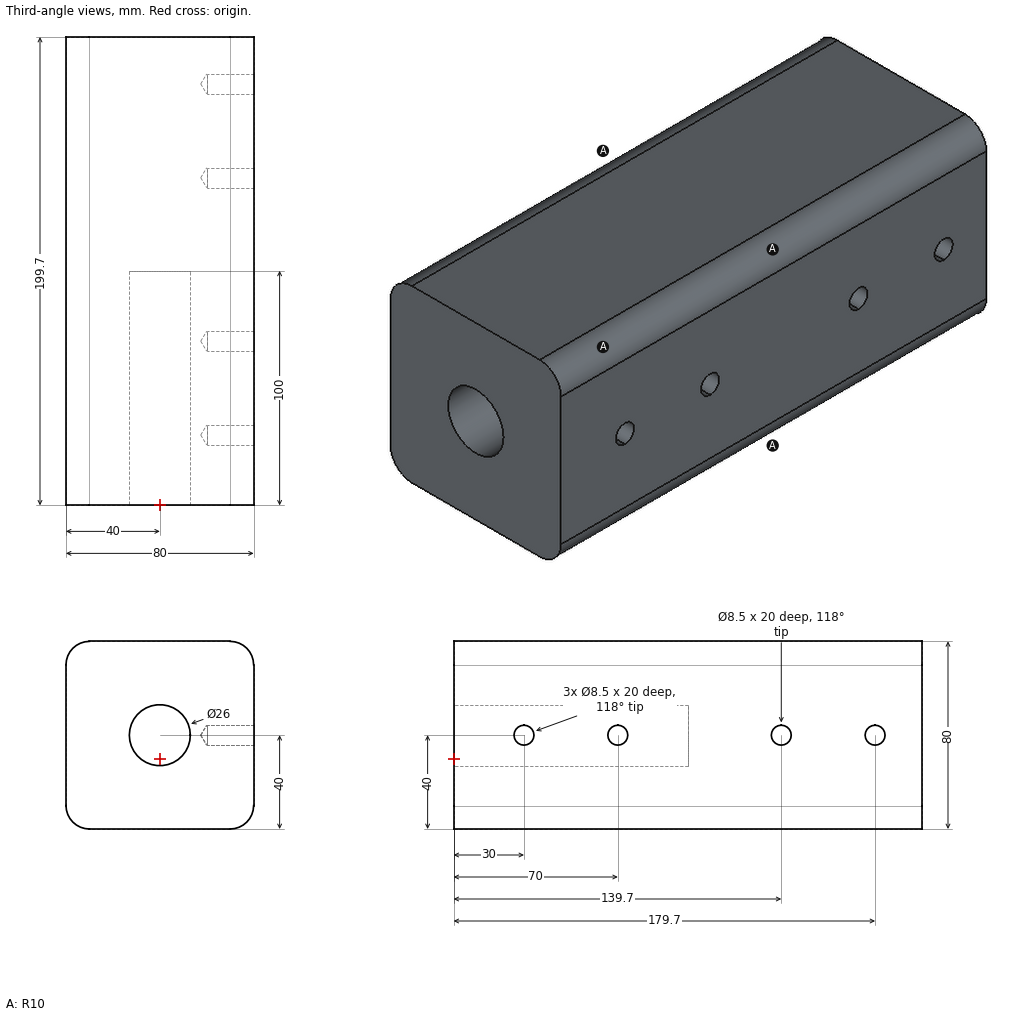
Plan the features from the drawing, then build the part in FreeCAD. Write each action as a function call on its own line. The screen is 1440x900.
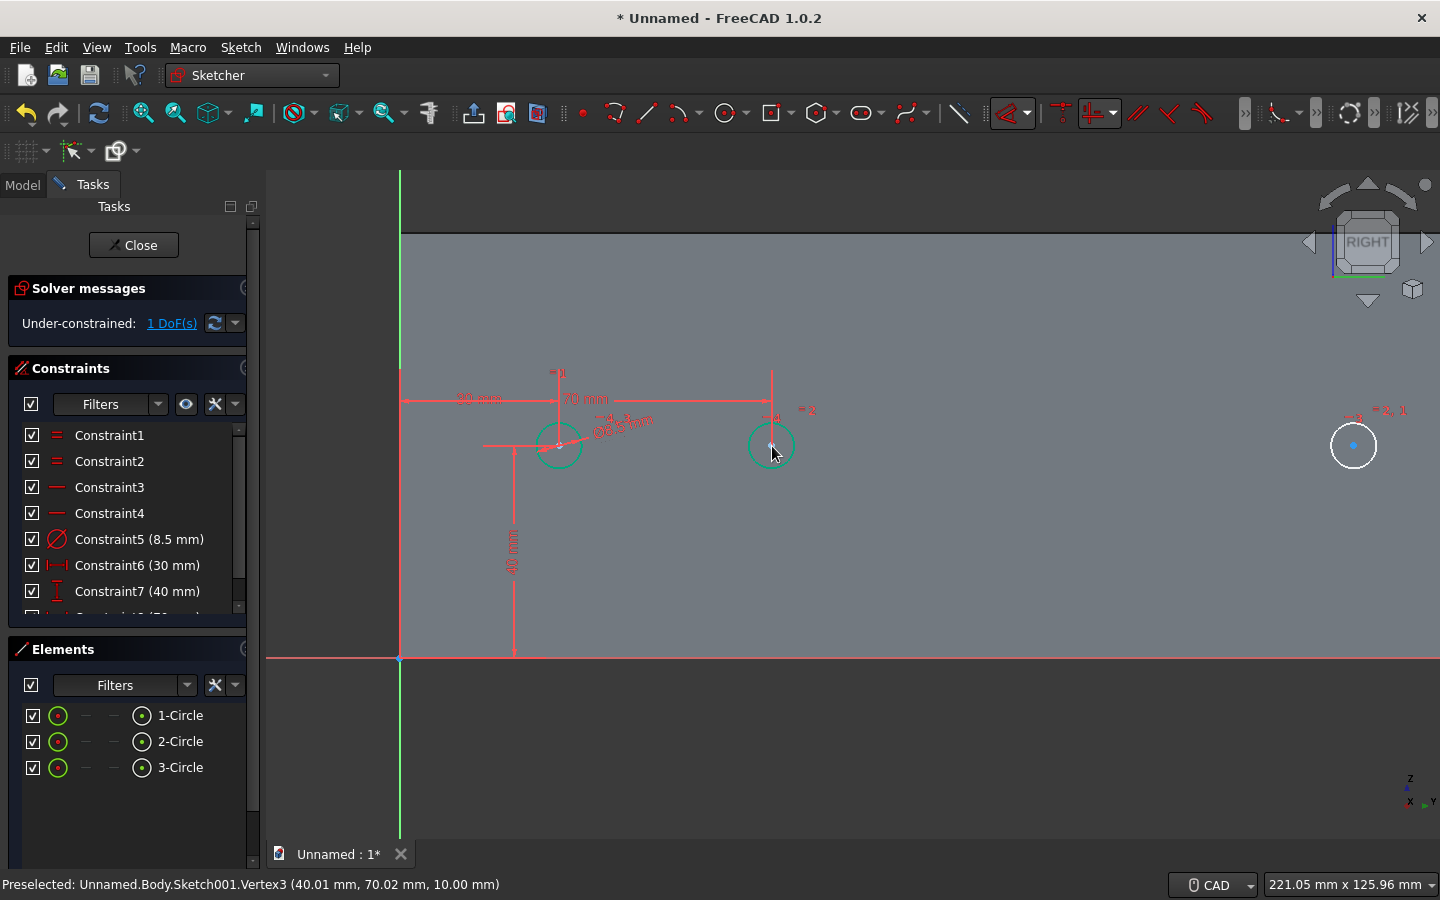
scroll(574, 431, down, 2)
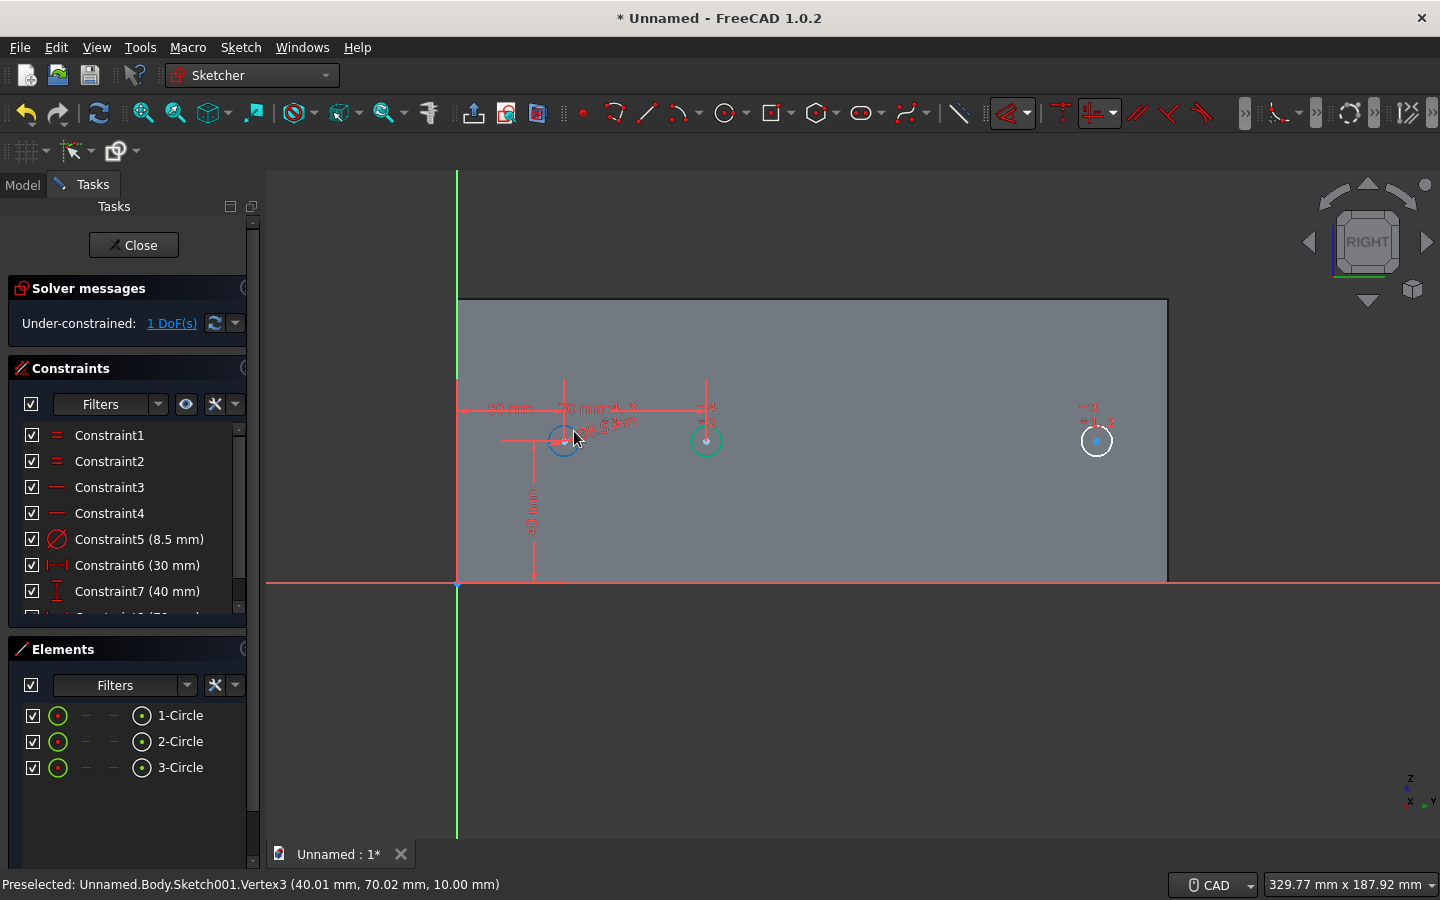
click(1097, 441)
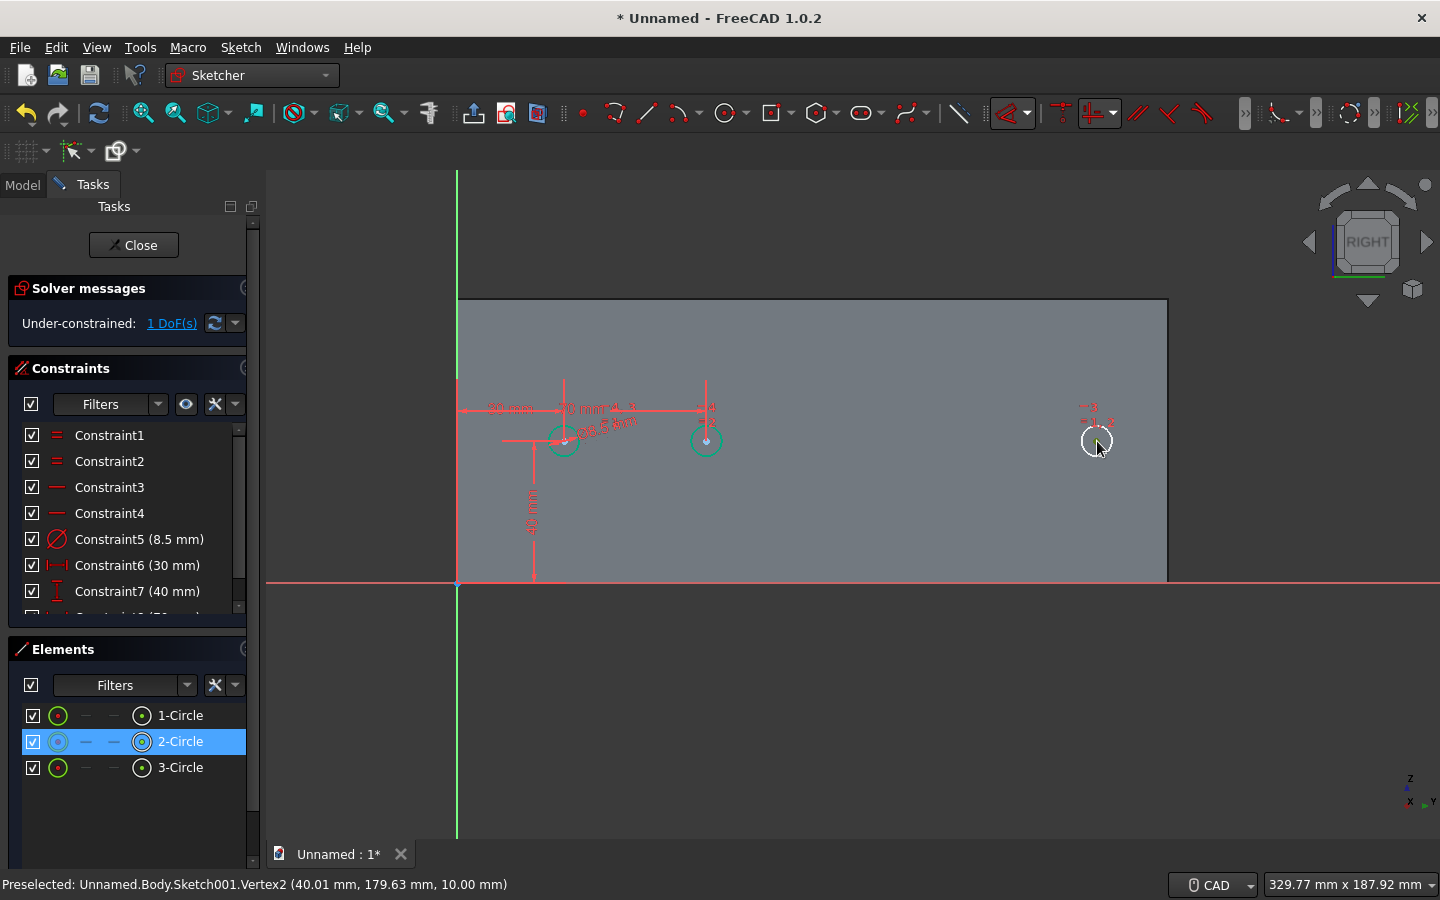
click(1030, 114)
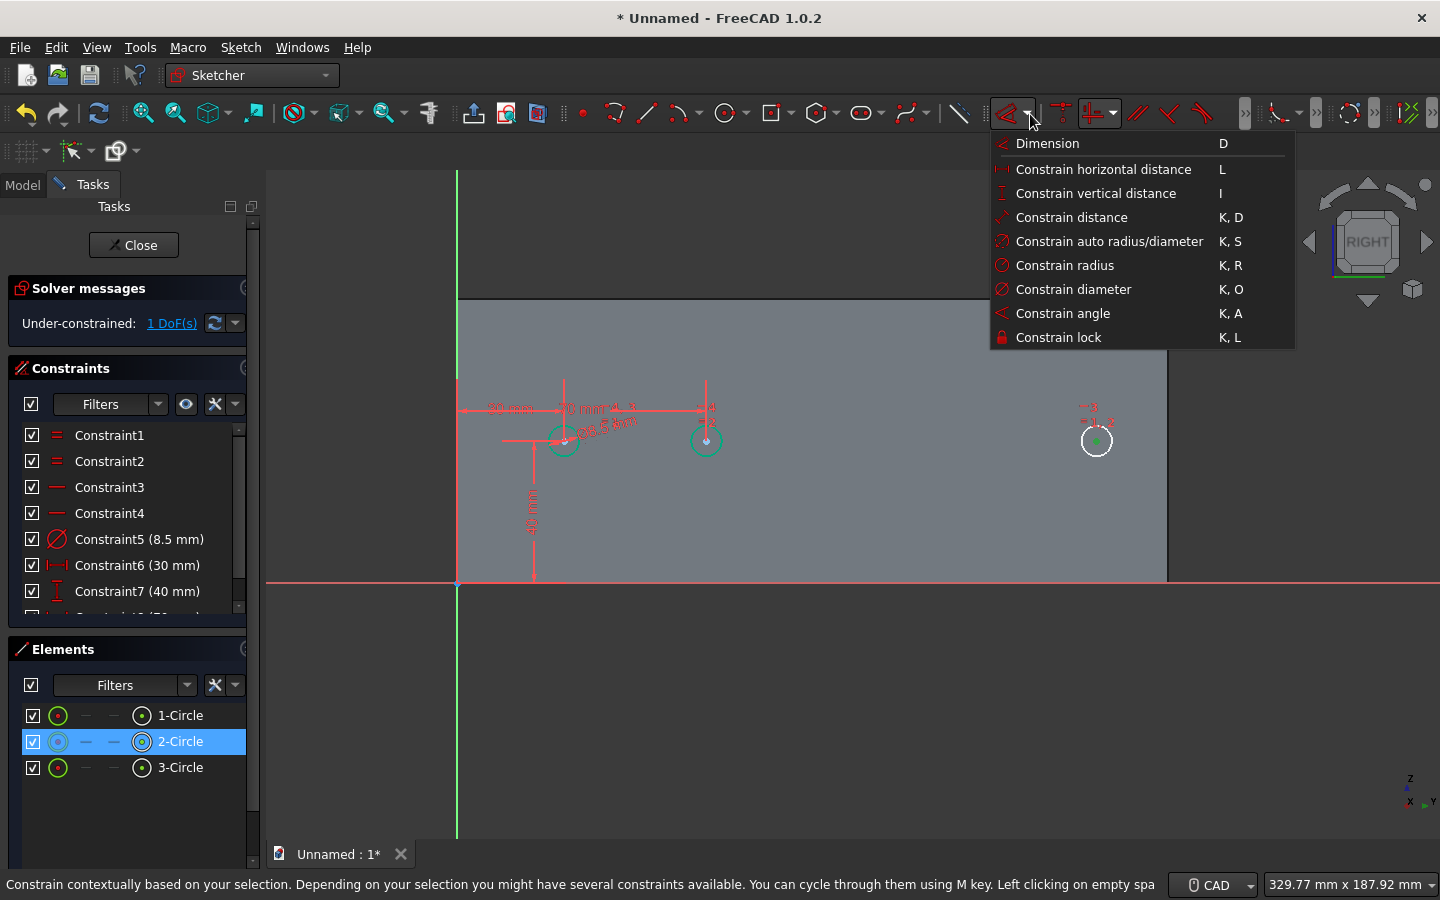
click(1143, 169)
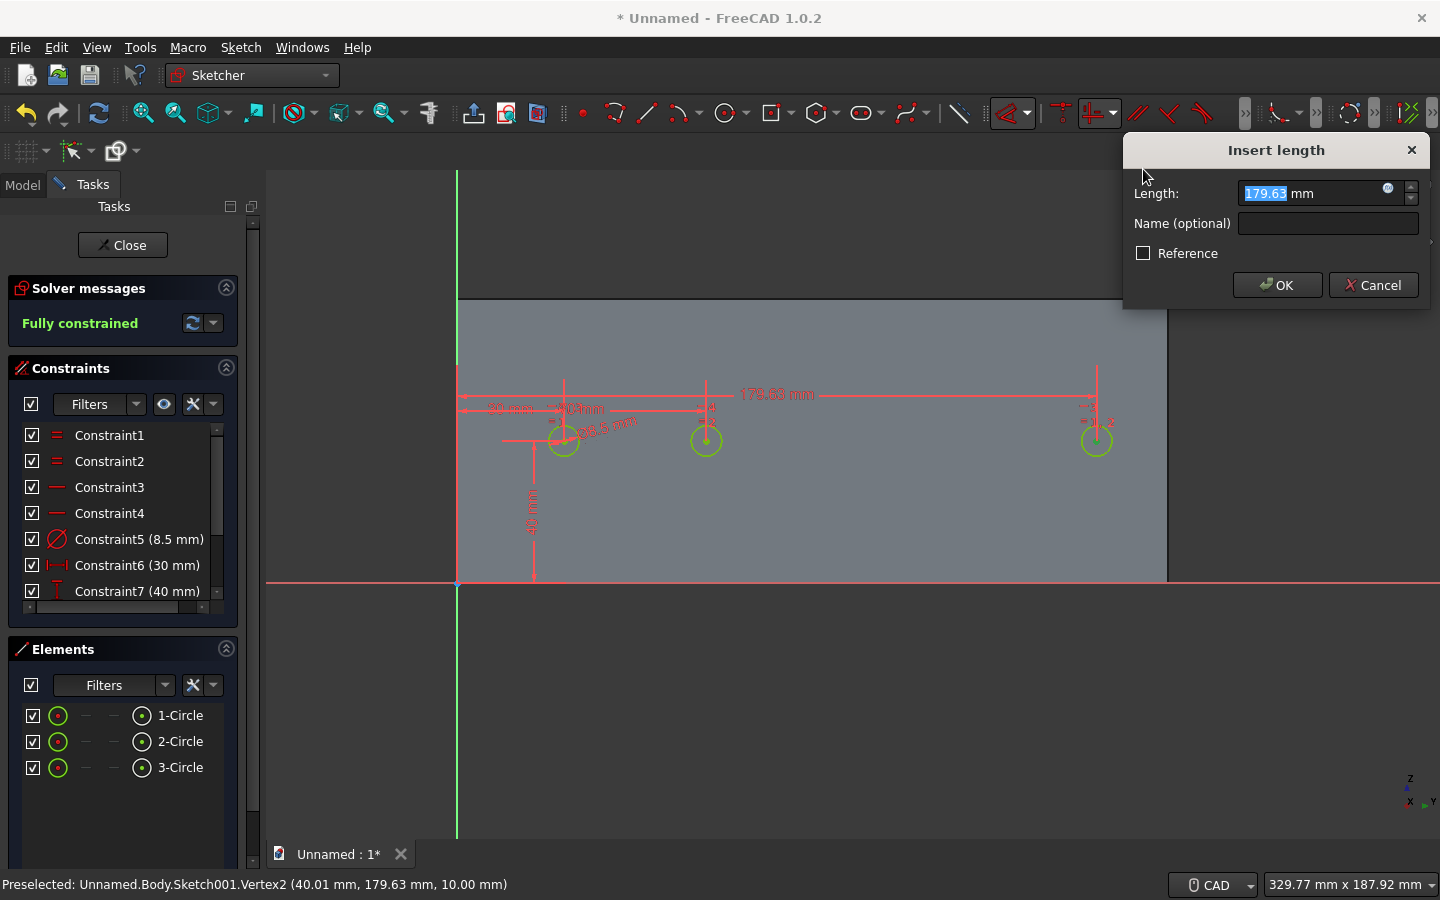
text(179.7)
key(Return)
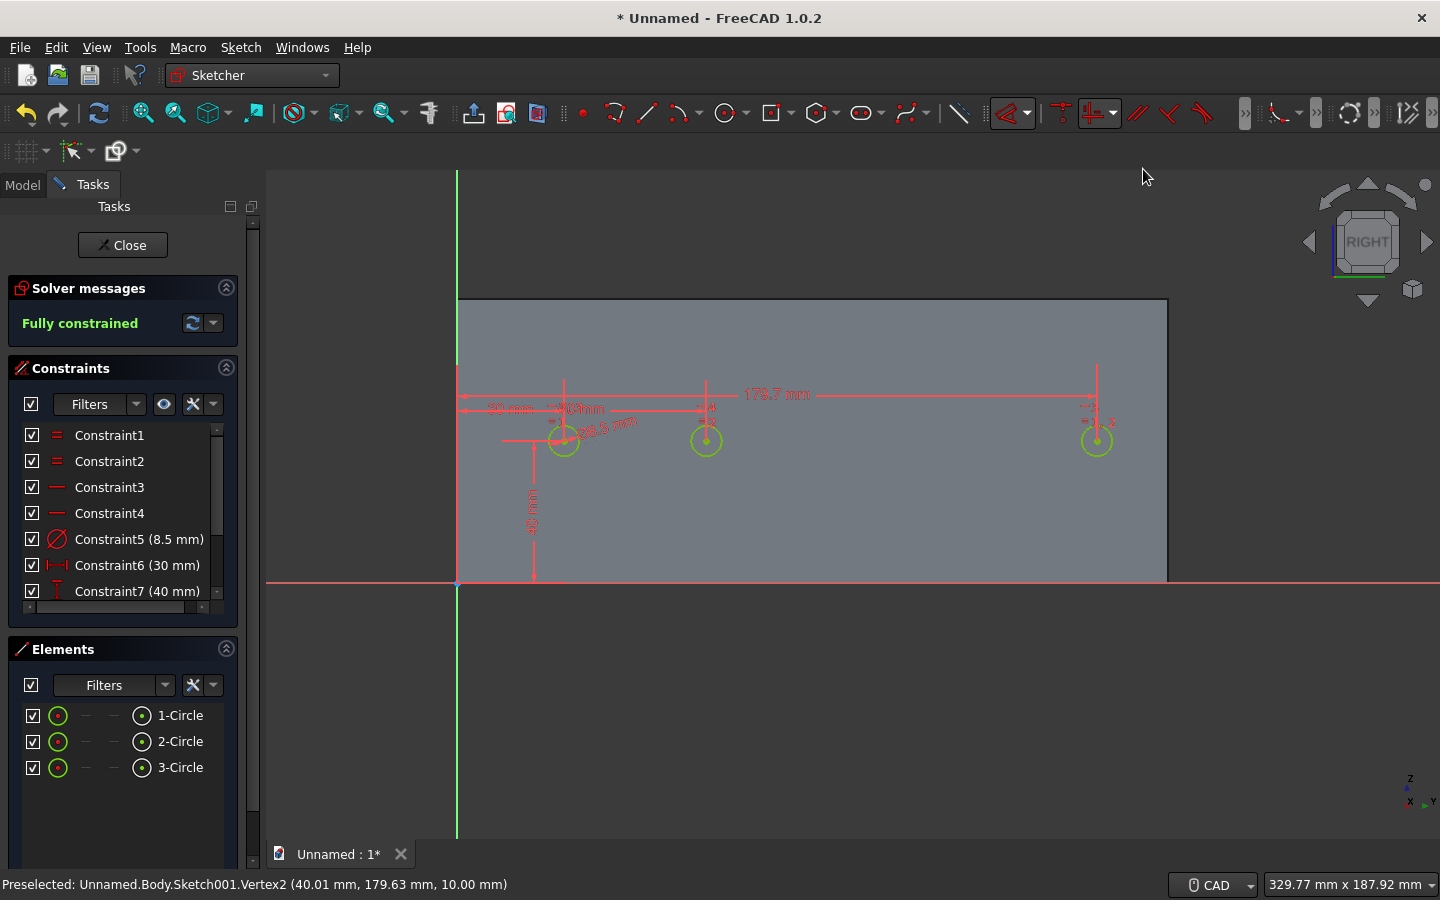
click(123, 245)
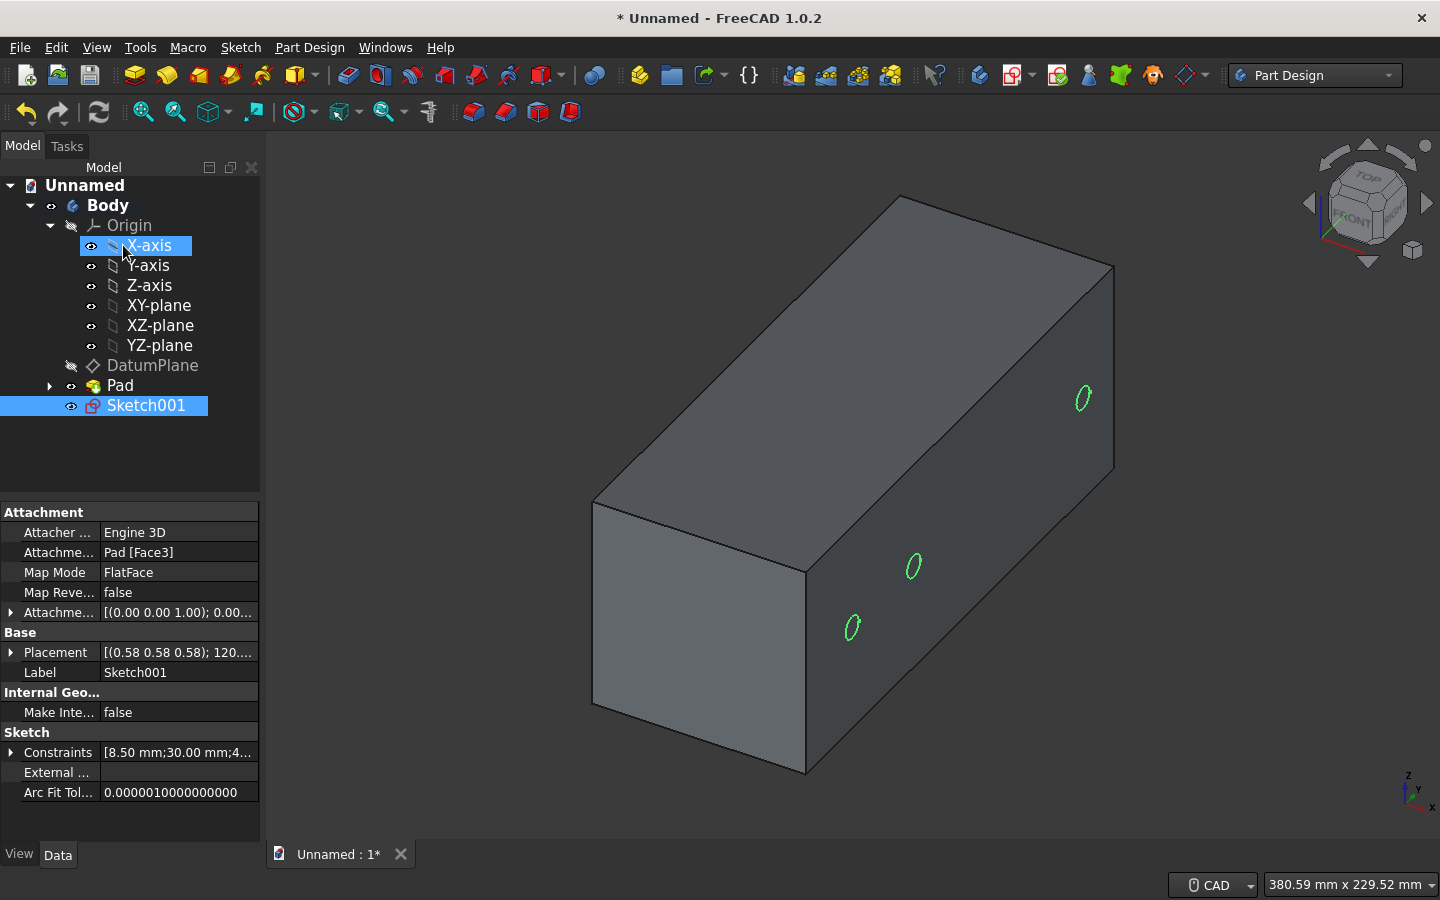
click(382, 76)